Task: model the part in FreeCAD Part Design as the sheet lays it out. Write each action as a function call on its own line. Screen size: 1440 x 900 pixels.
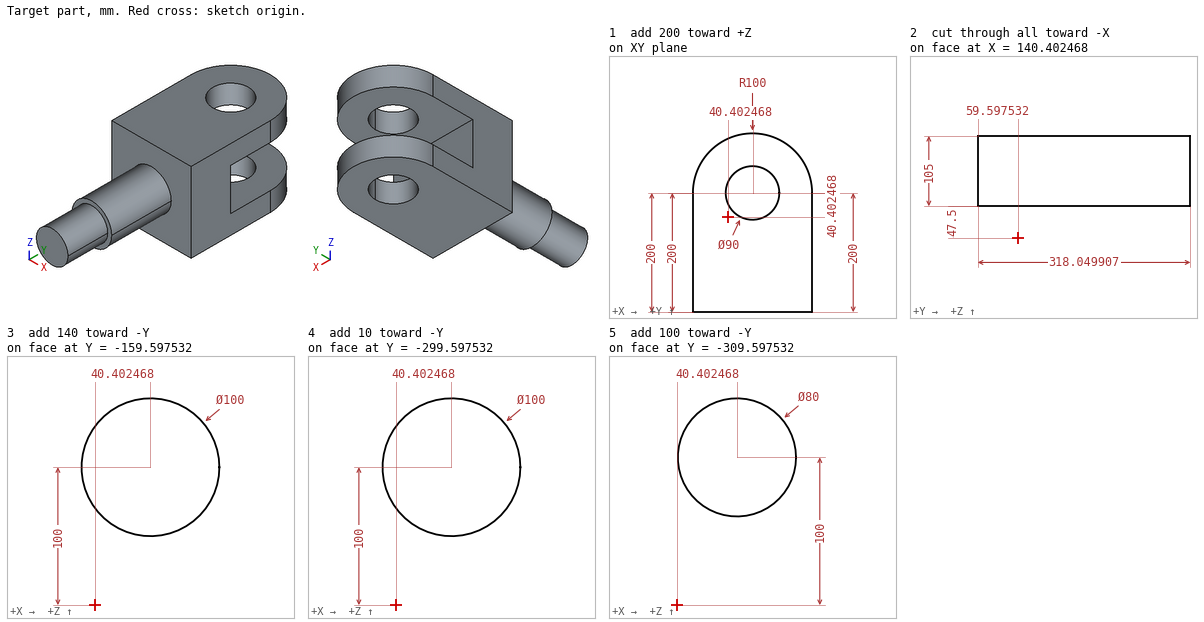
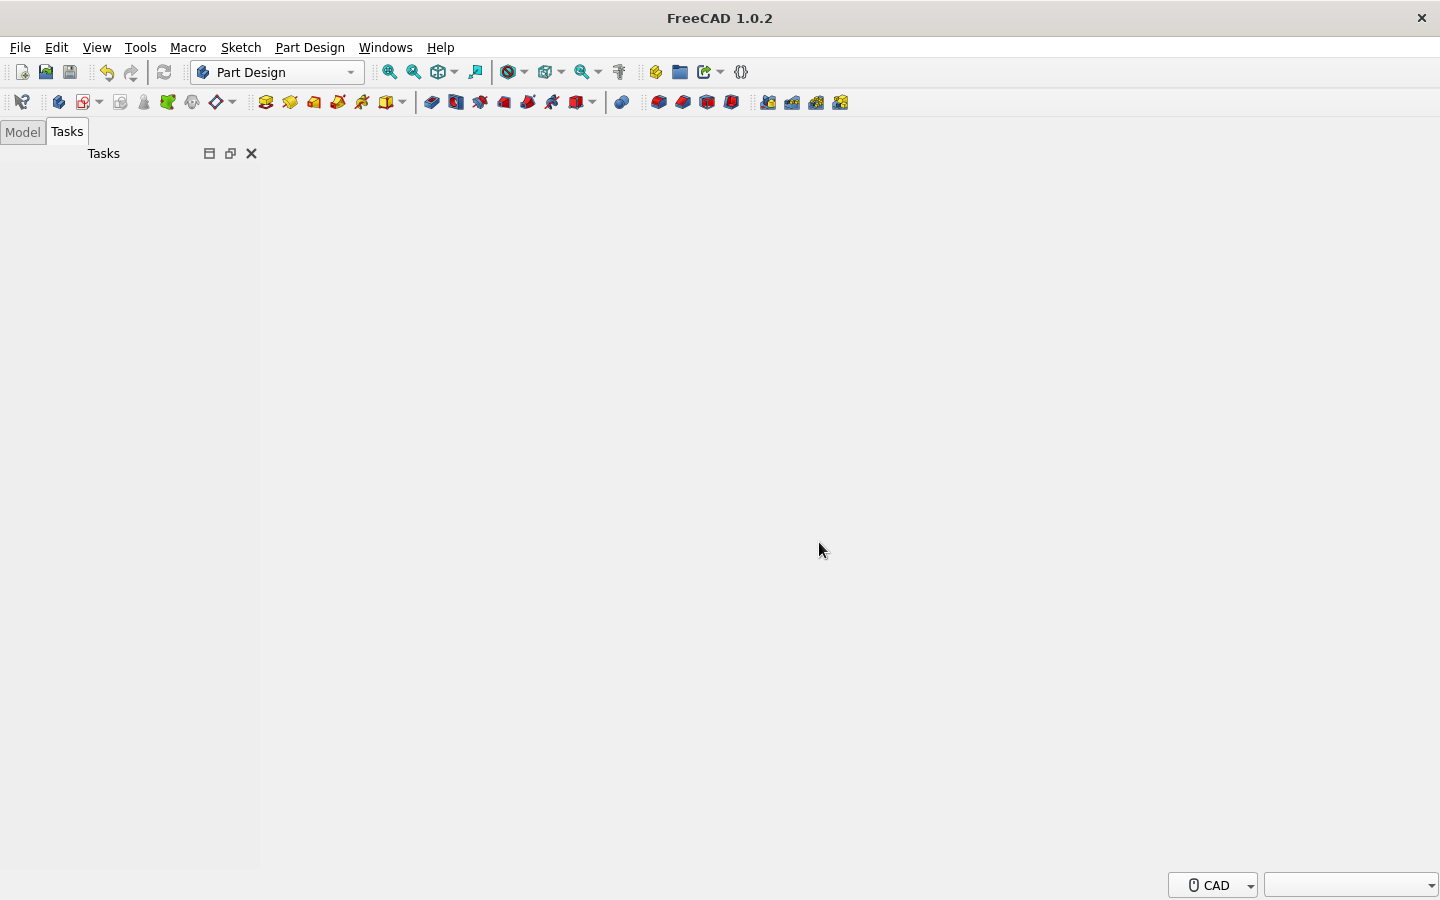
key(ctrl+n)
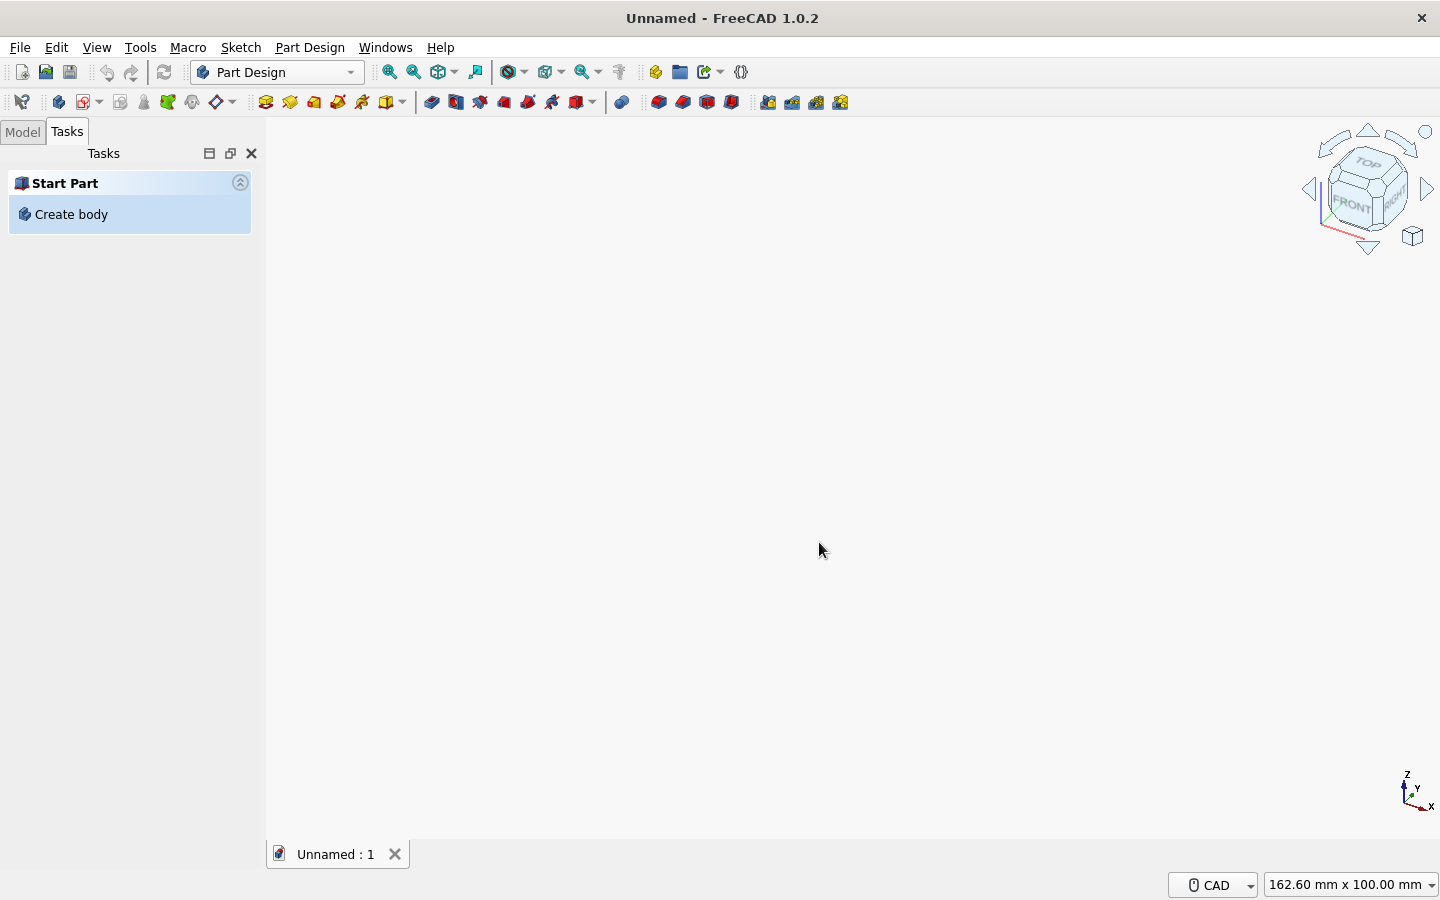
click(84, 102)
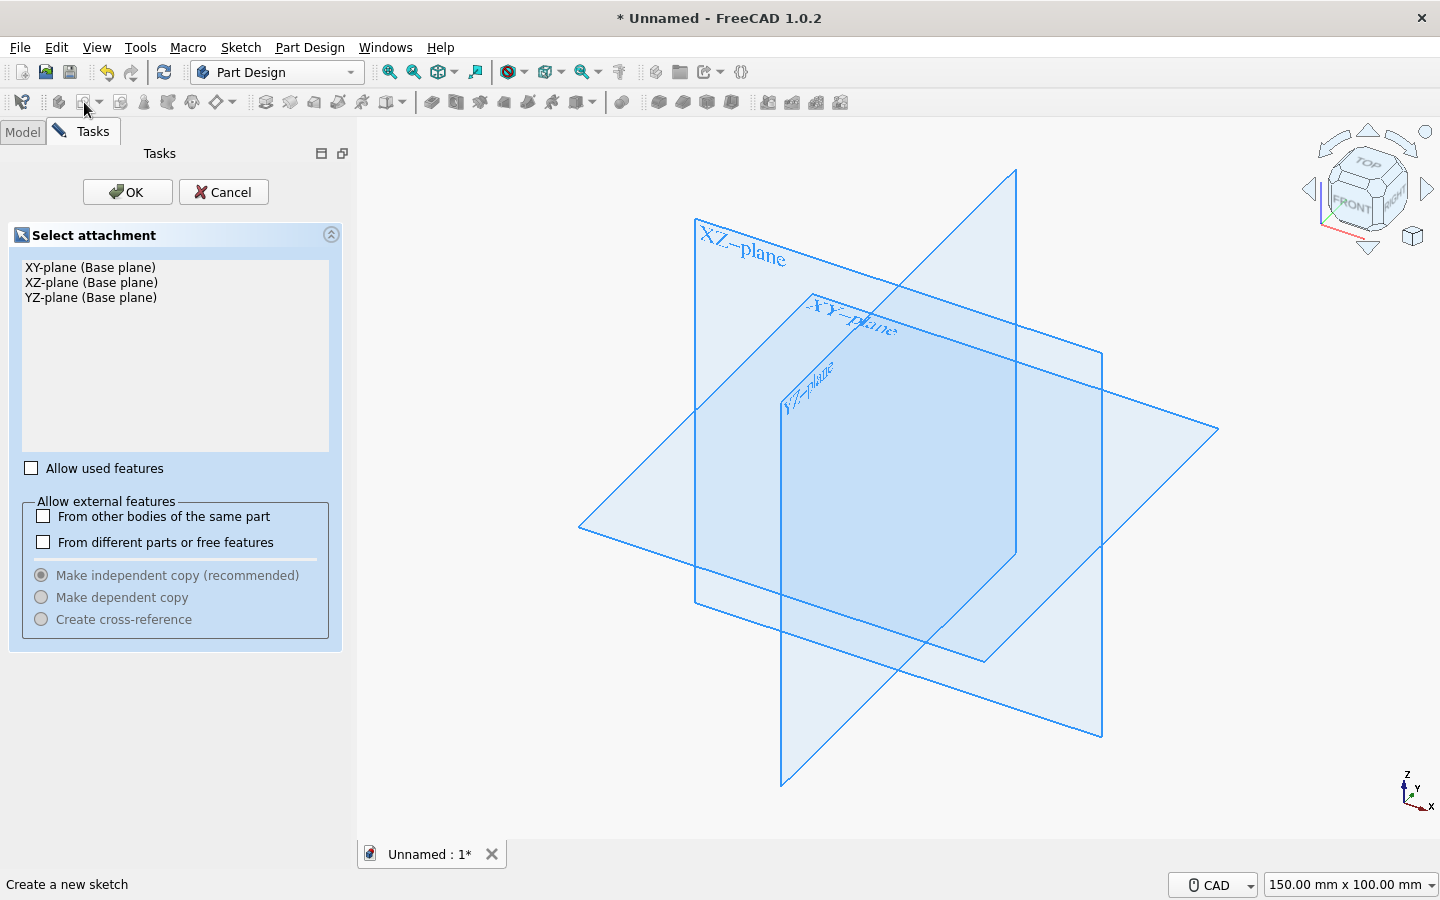
click(82, 268)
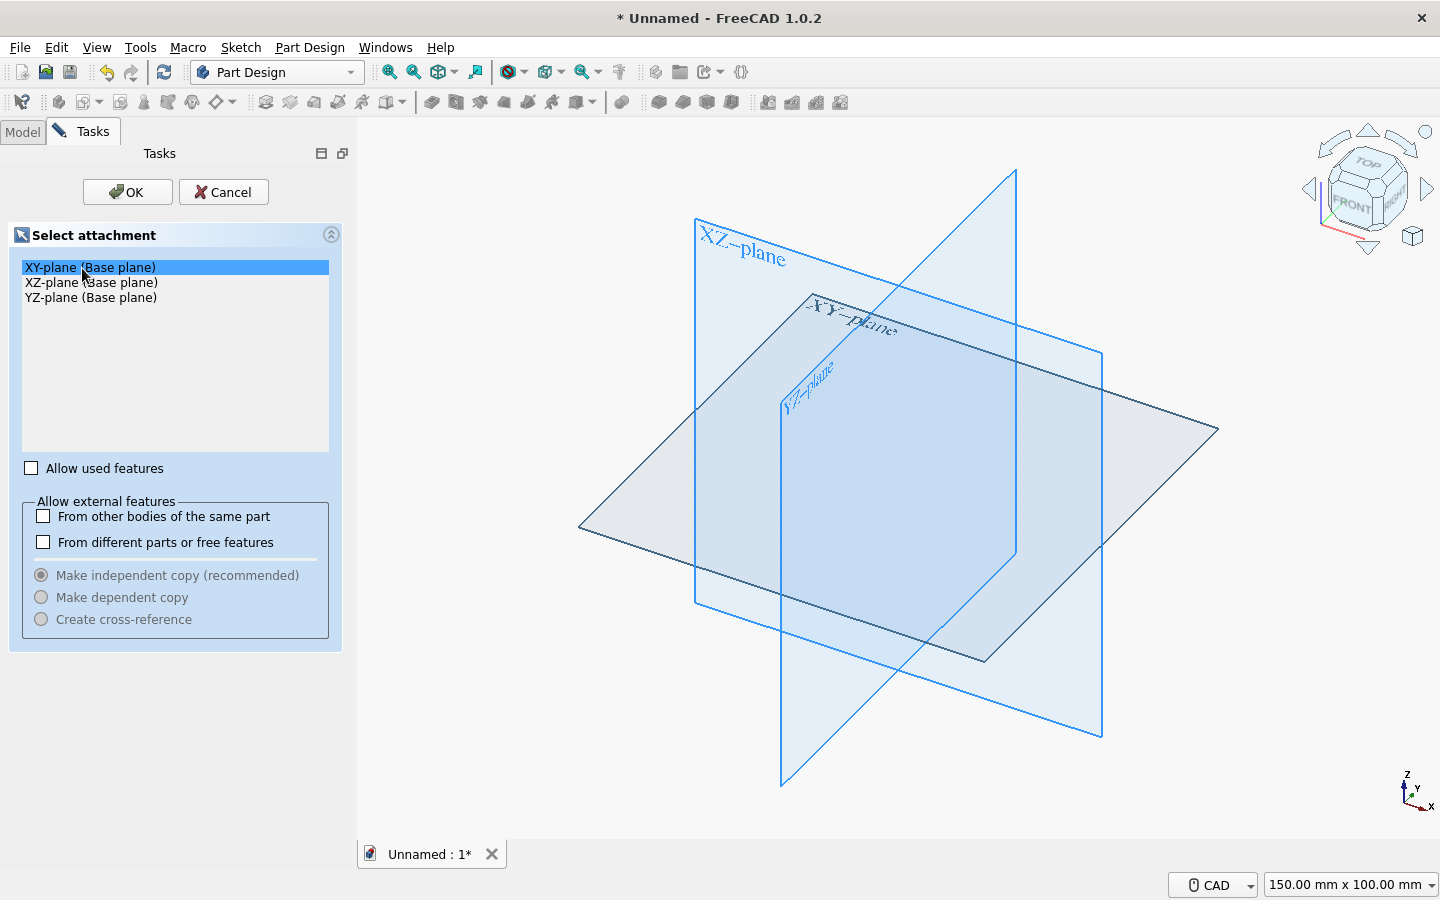
click(128, 192)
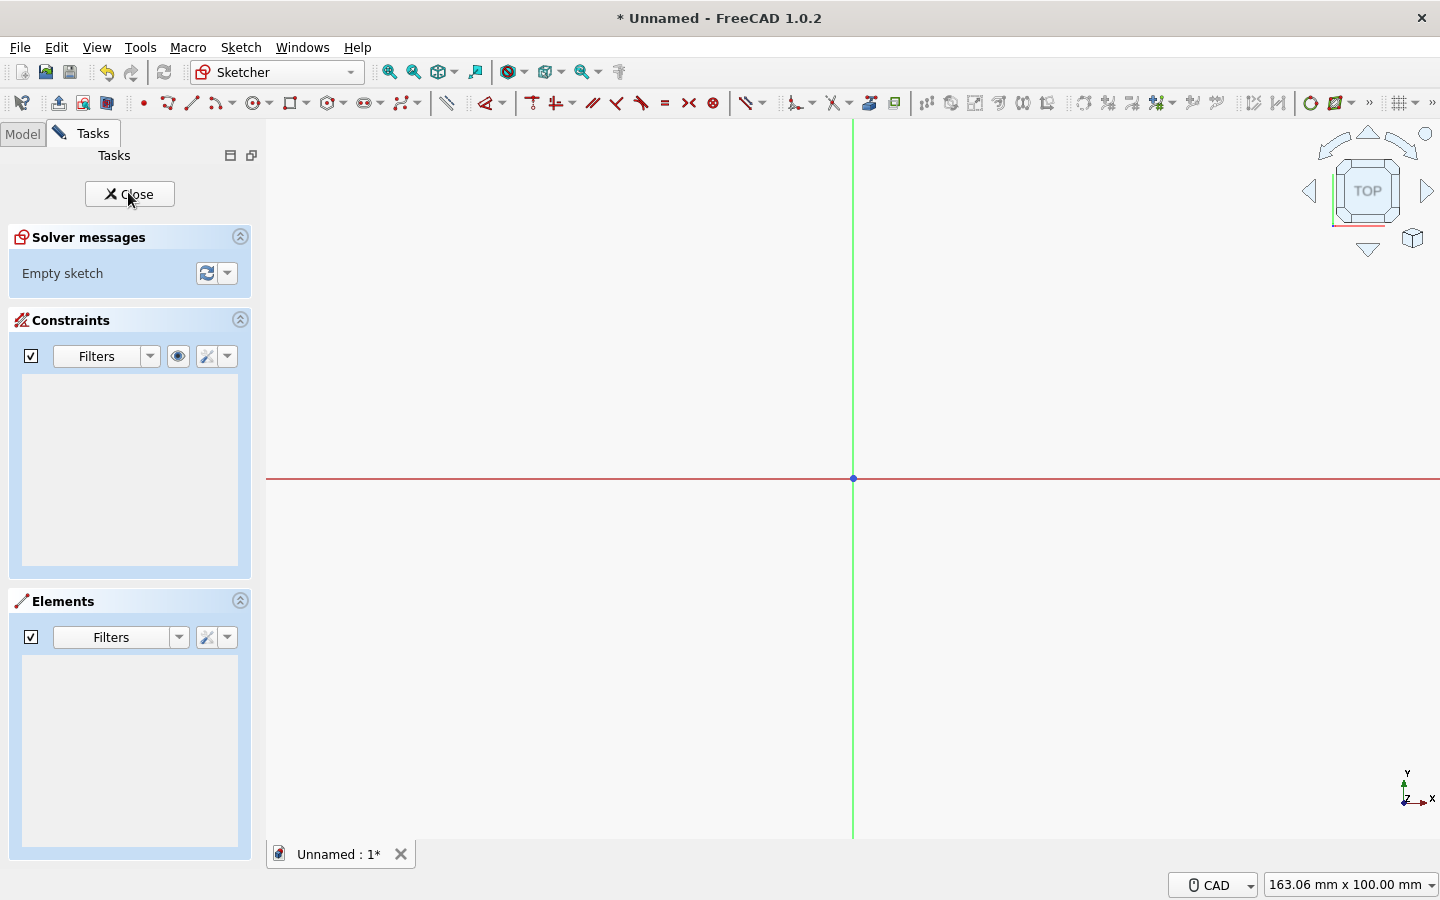
scroll(694, 462, down, 8)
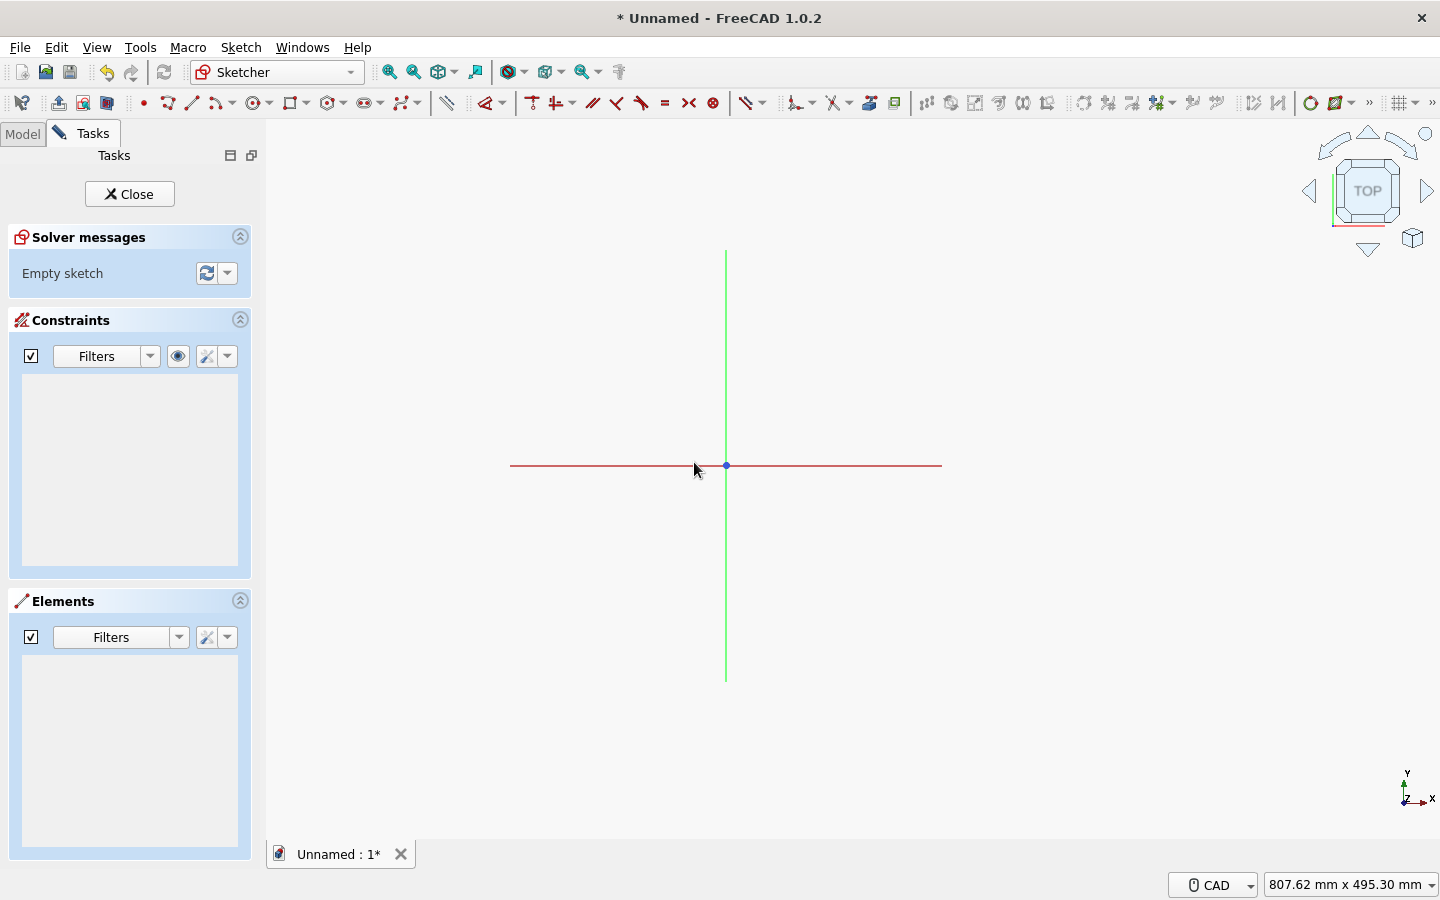
click(168, 104)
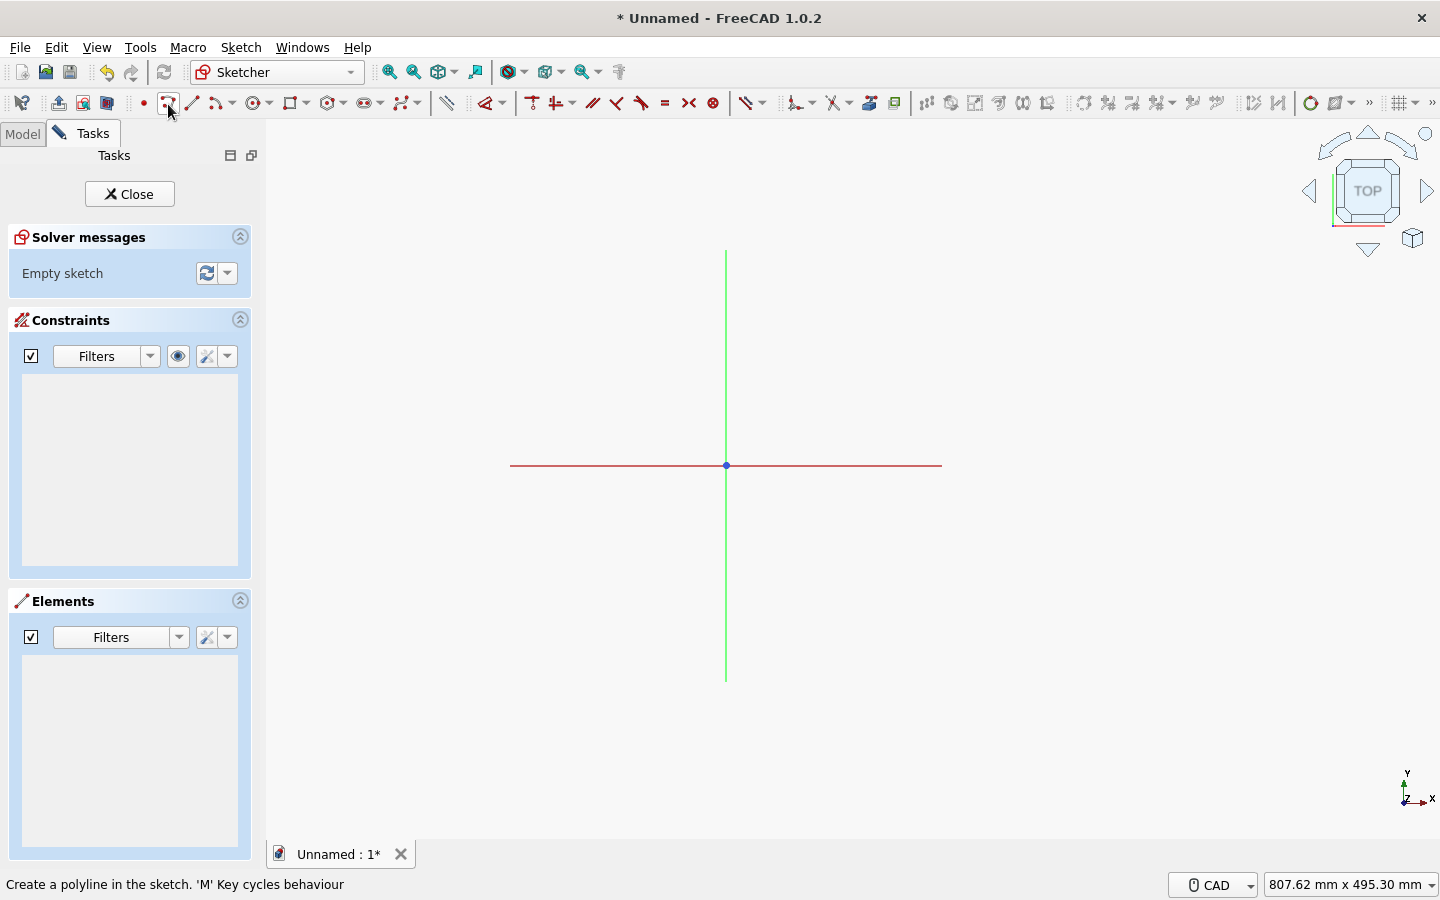
click(640, 407)
click(640, 698)
click(930, 698)
click(930, 407)
right_click(930, 407)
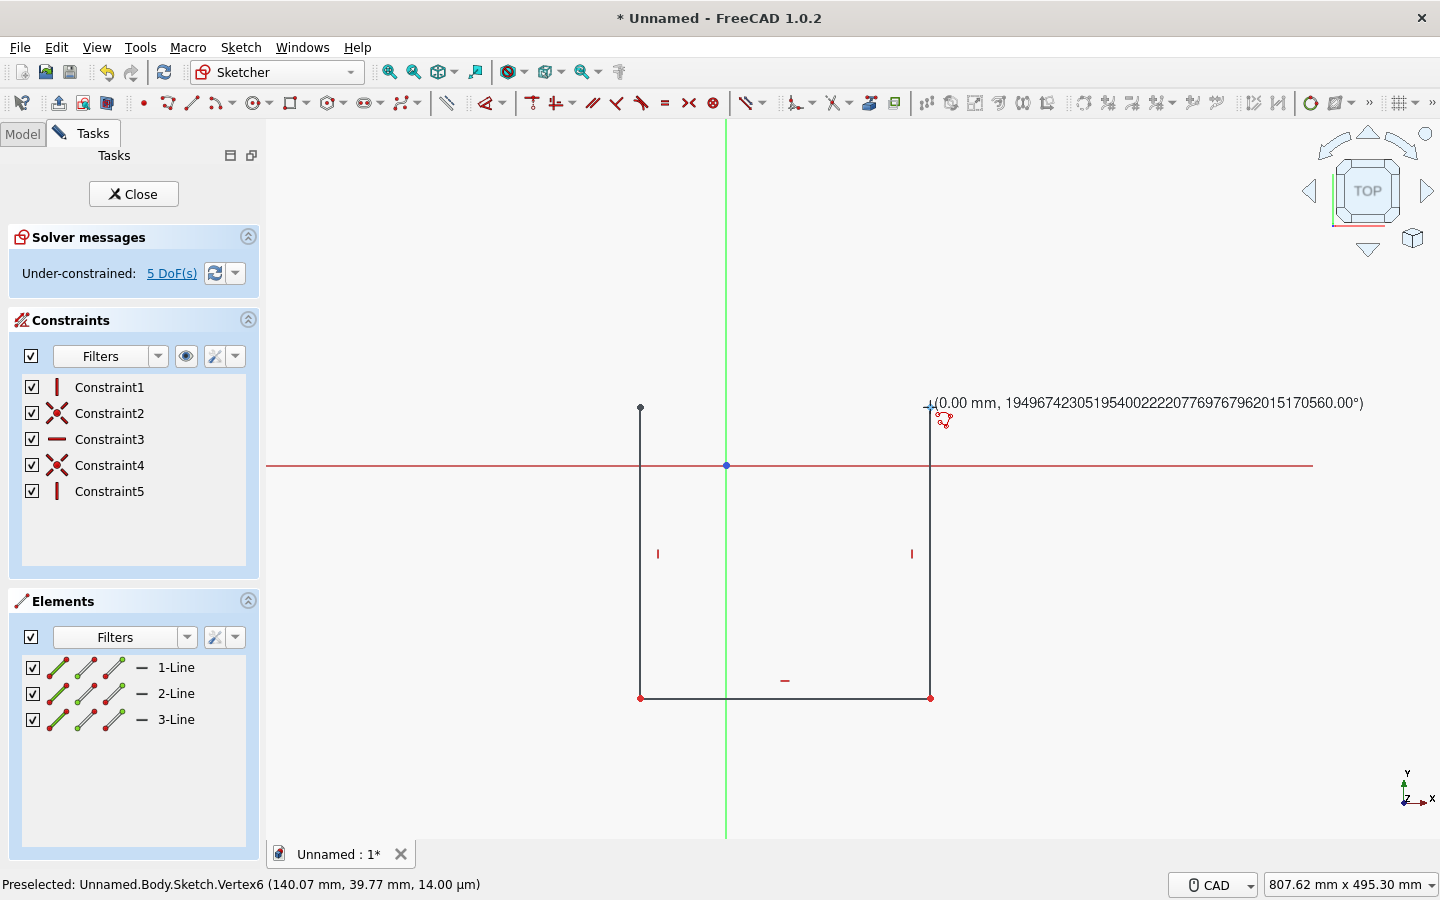
click(234, 104)